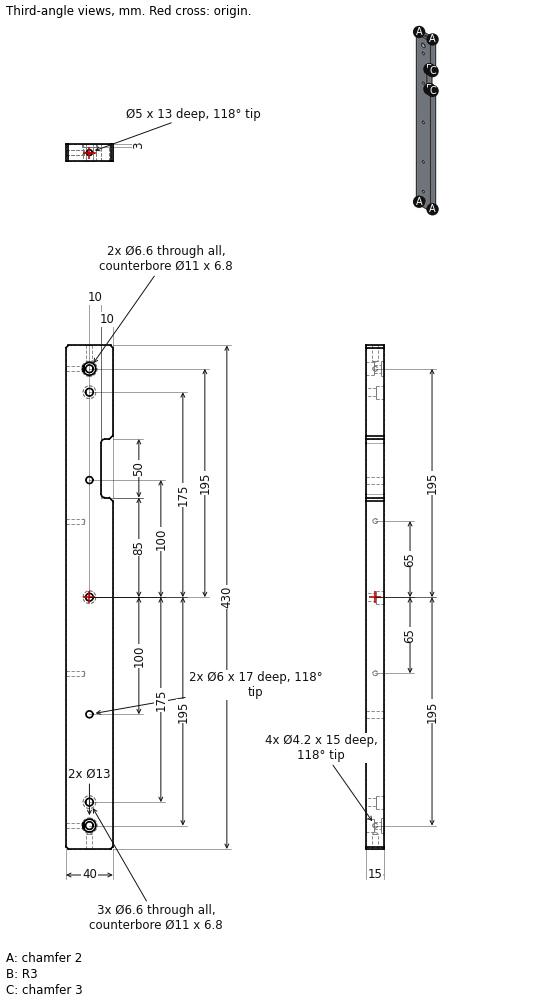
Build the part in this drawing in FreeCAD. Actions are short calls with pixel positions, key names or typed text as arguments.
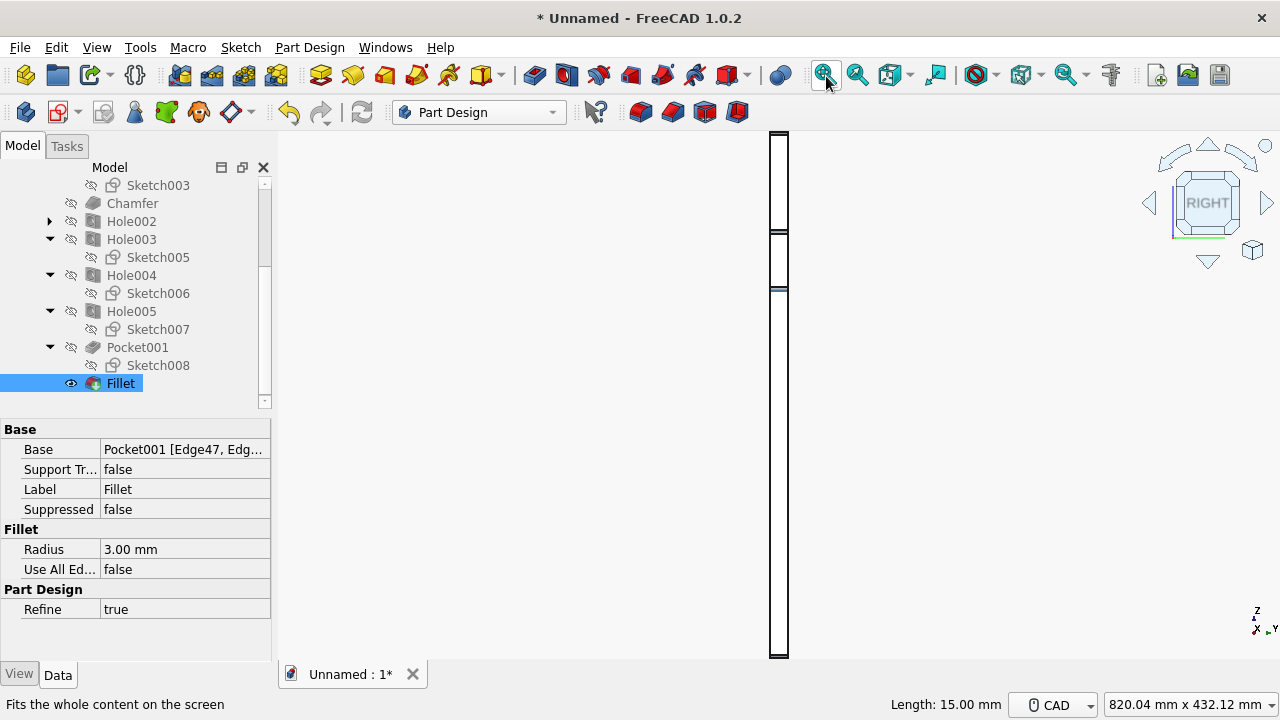
click(779, 229, ctrl)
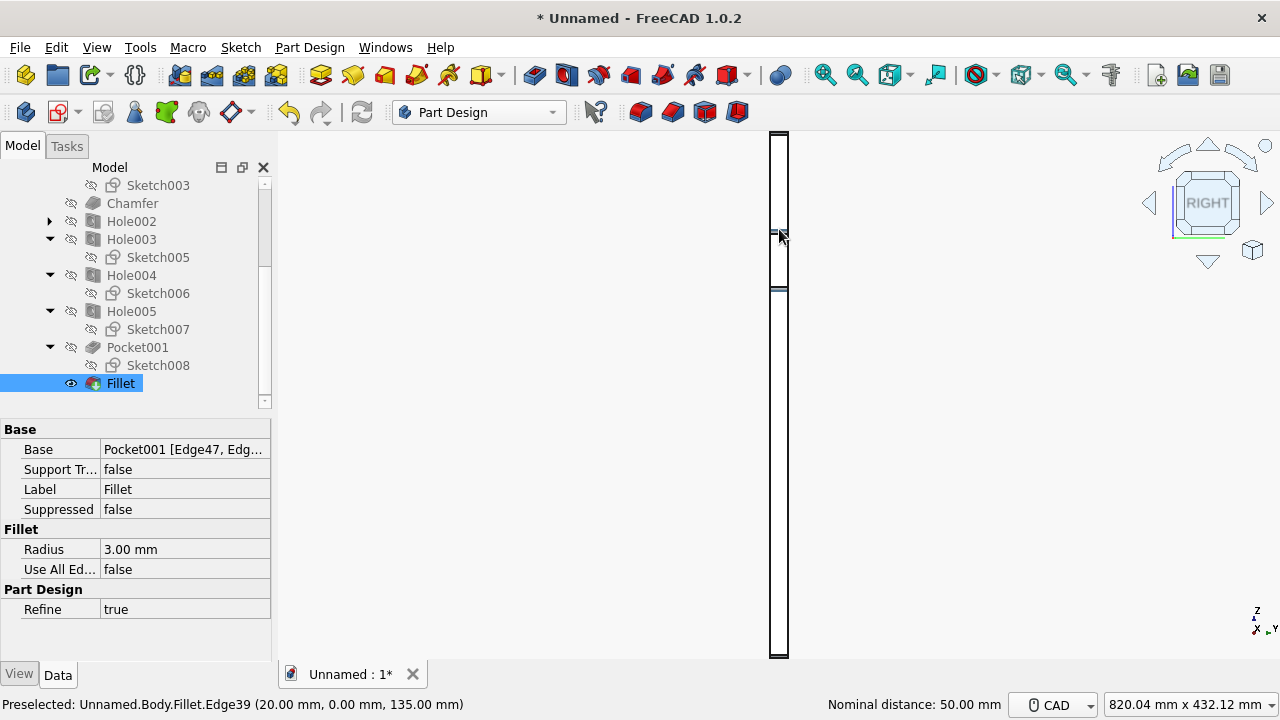
click(674, 112)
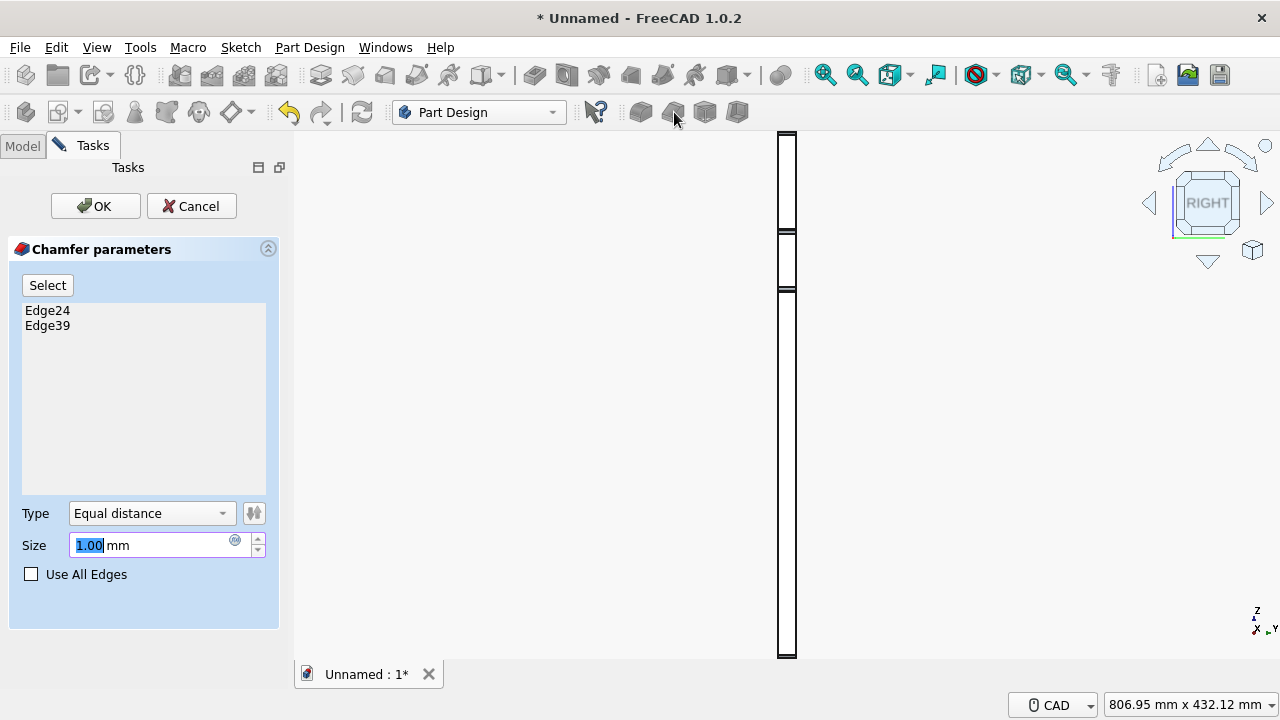
text(3)
key(Tab)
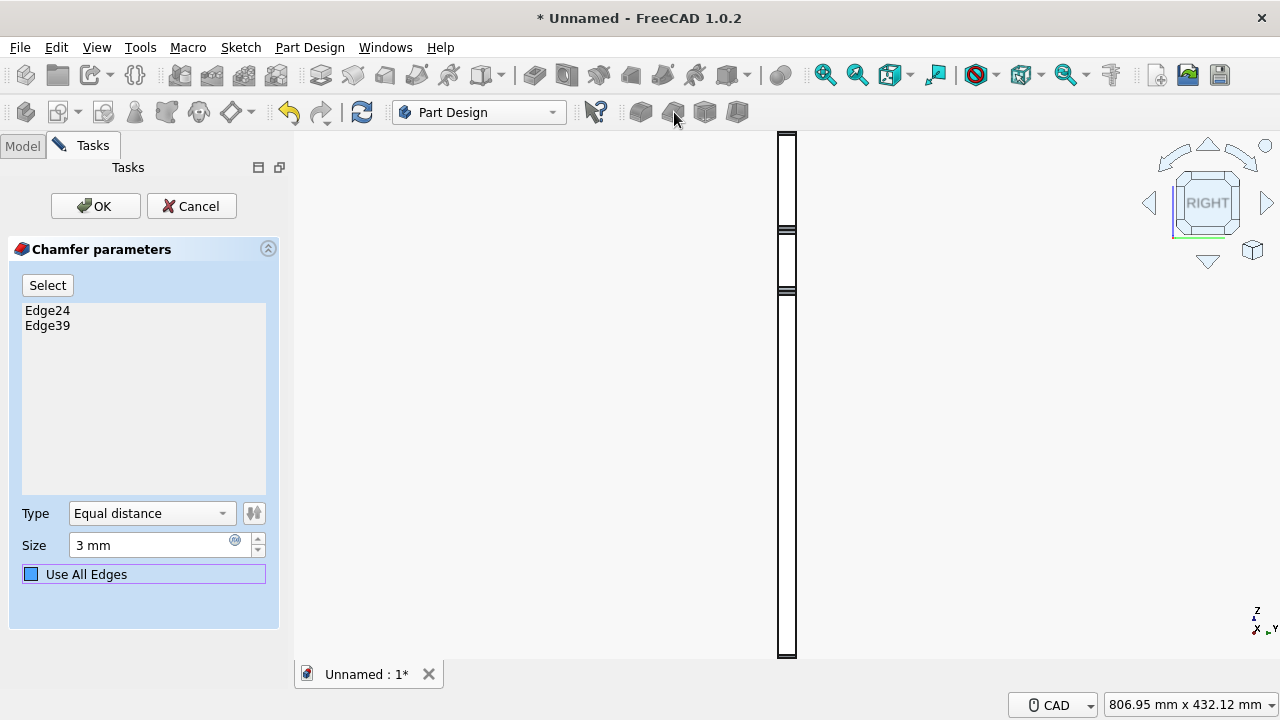
click(96, 206)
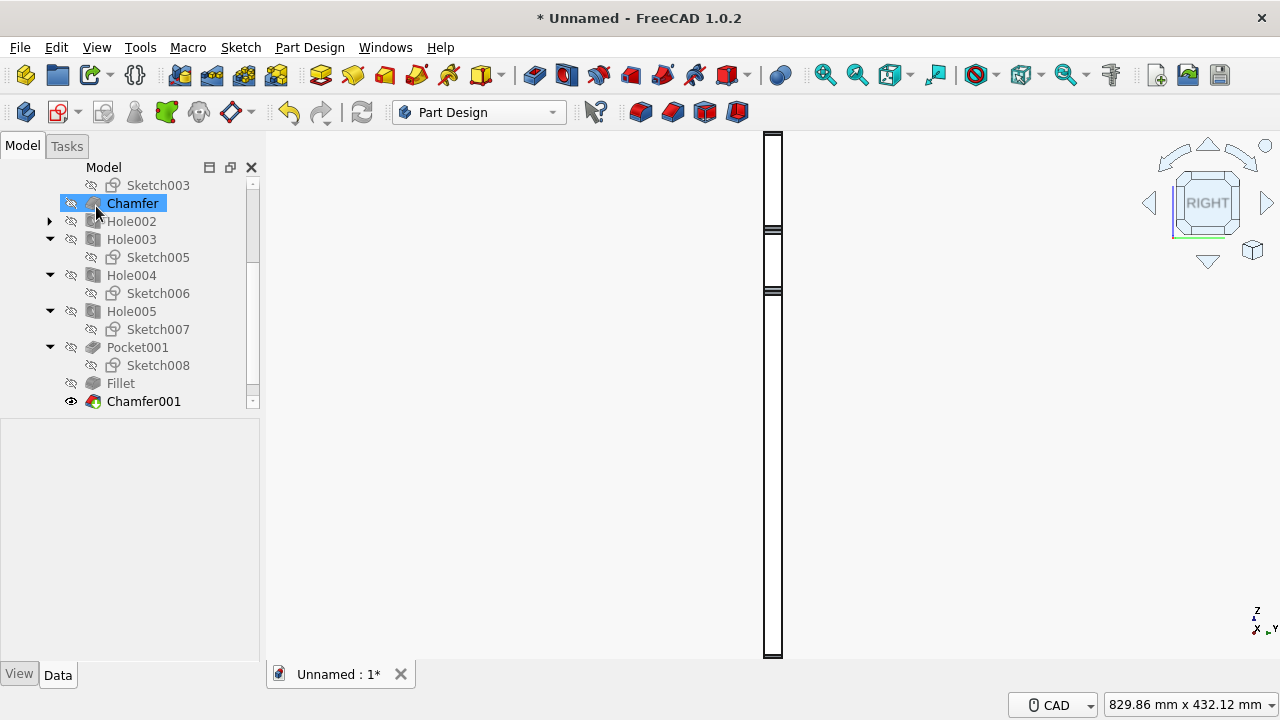
key(0)